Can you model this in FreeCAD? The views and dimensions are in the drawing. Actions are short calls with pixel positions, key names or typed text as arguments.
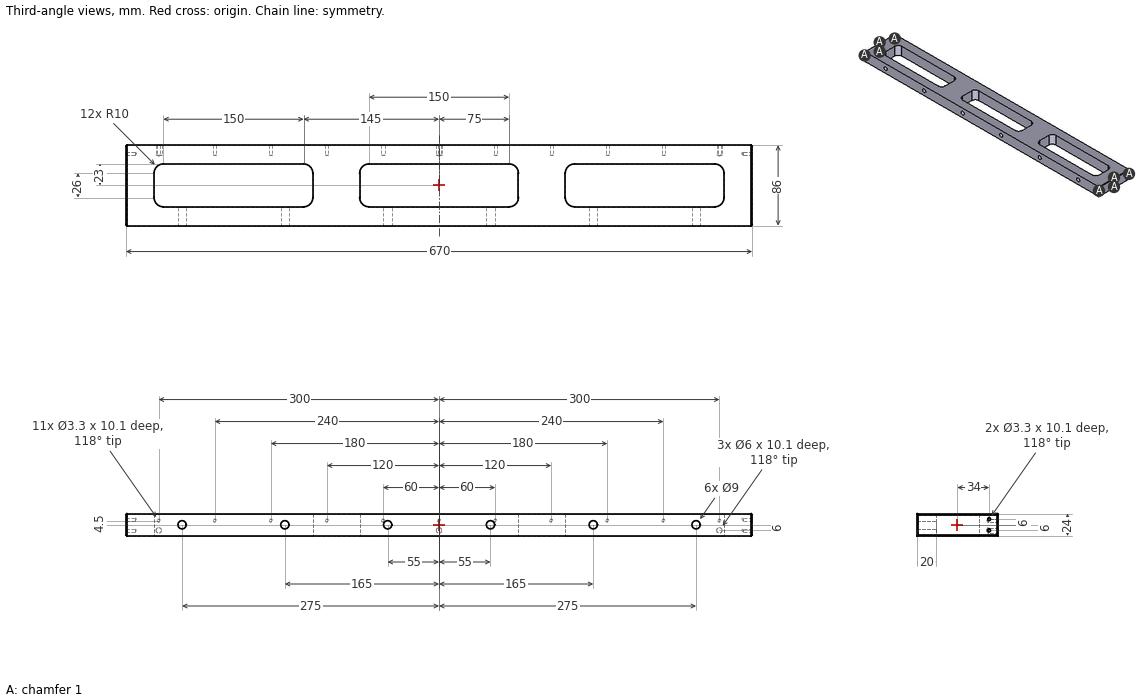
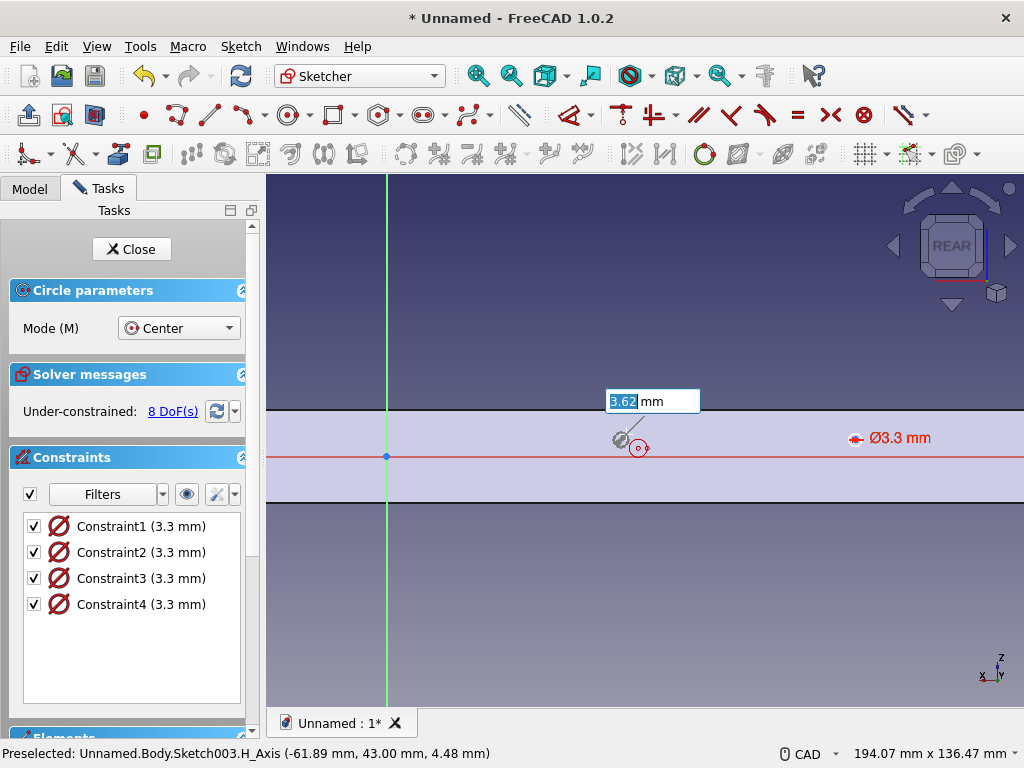
text(3.3)
key(Return)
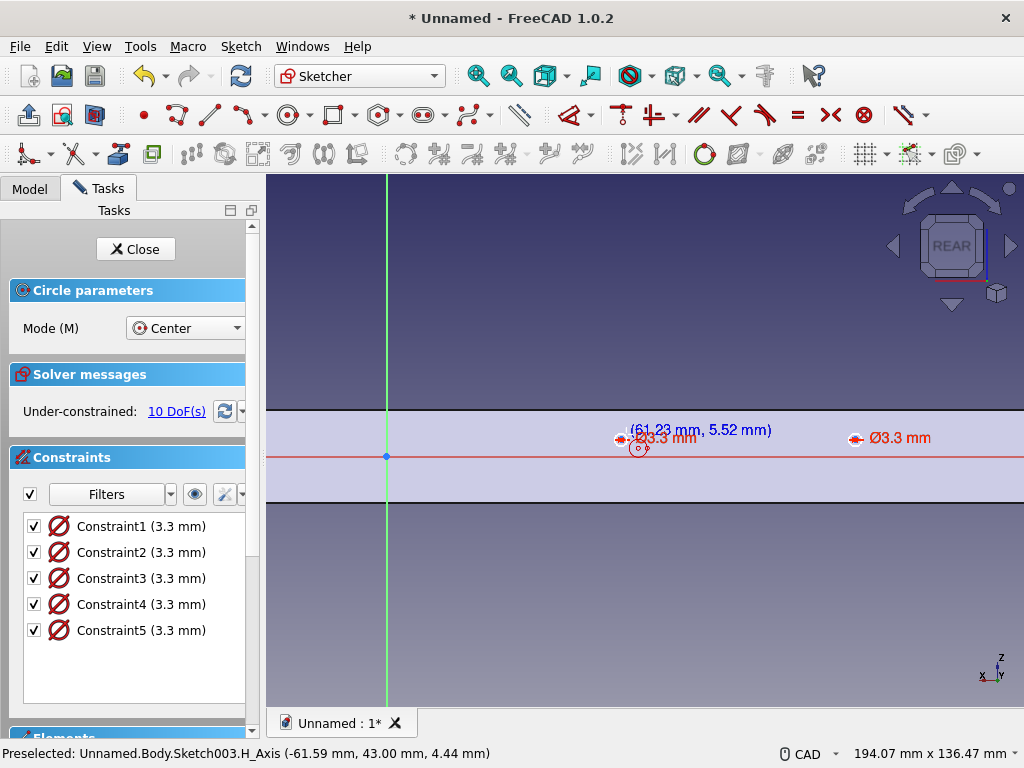
scroll(387, 439, up, 7)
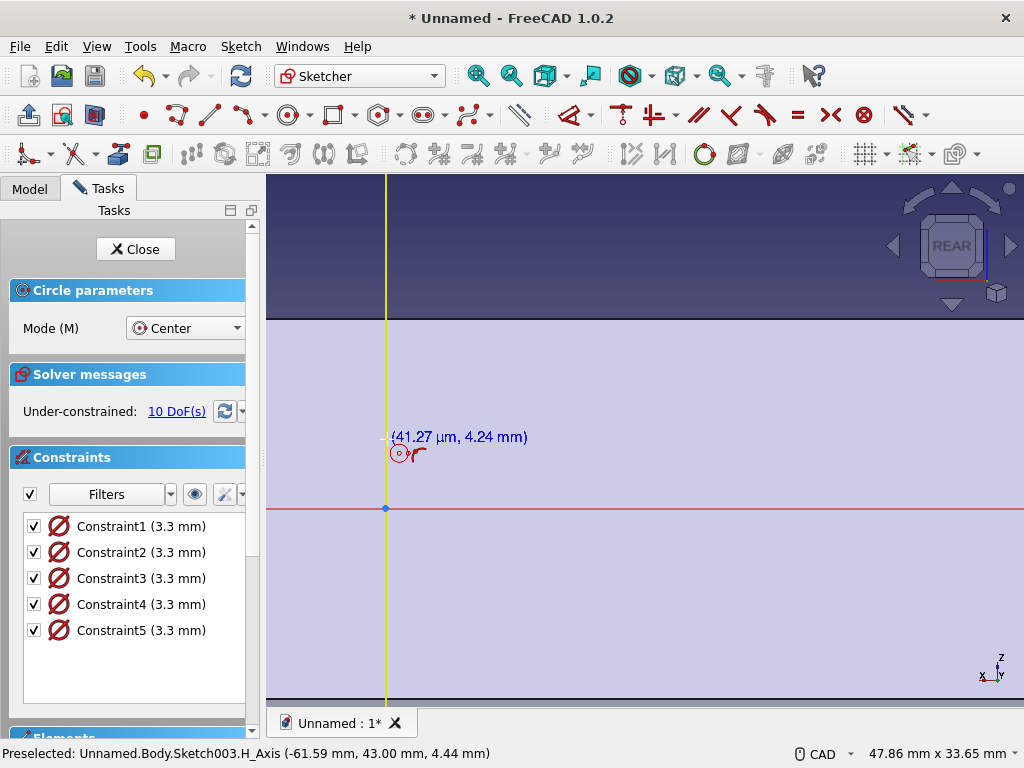
scroll(586, 439, down, 15)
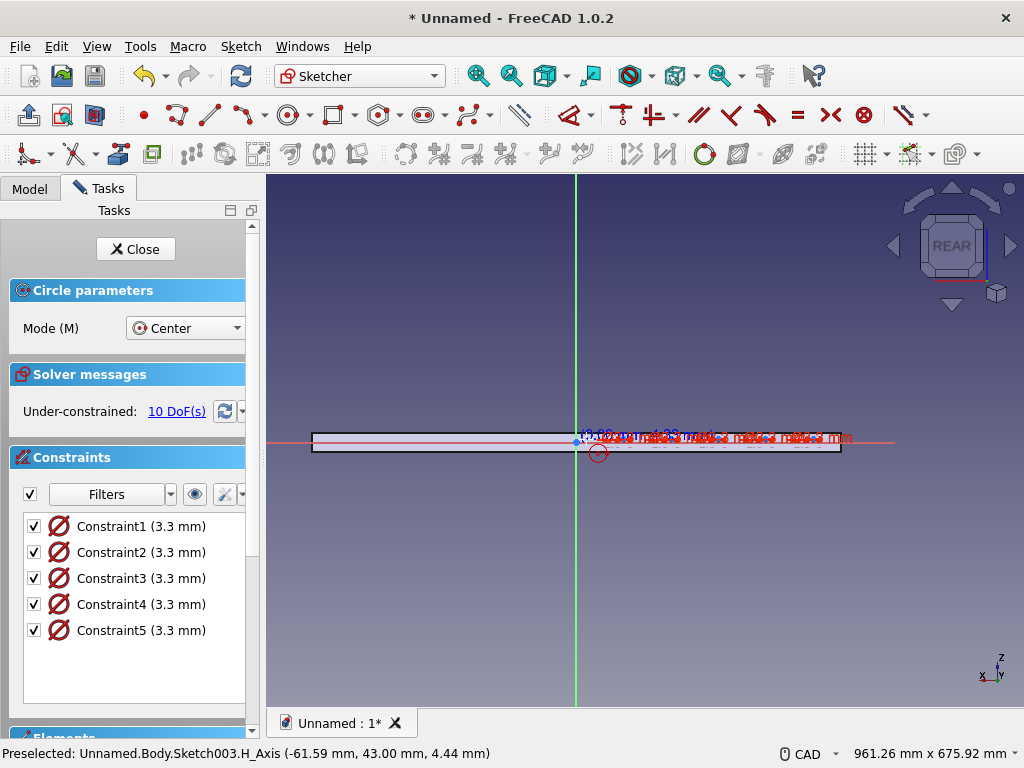
scroll(576, 439, up, 8)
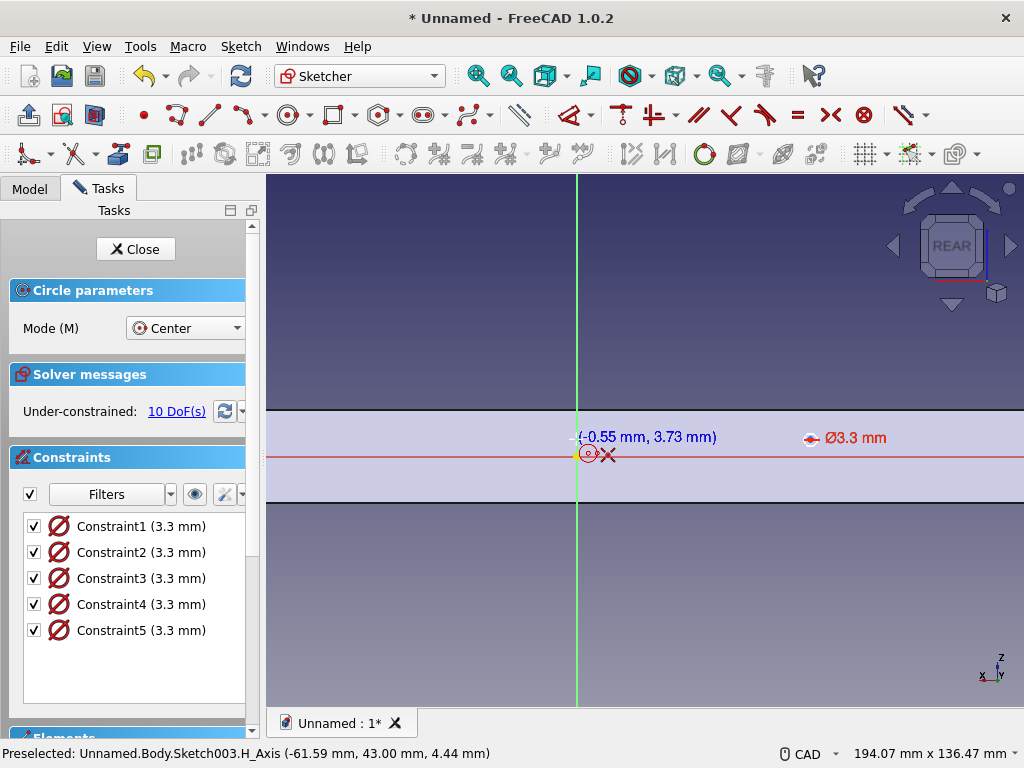
click(577, 439)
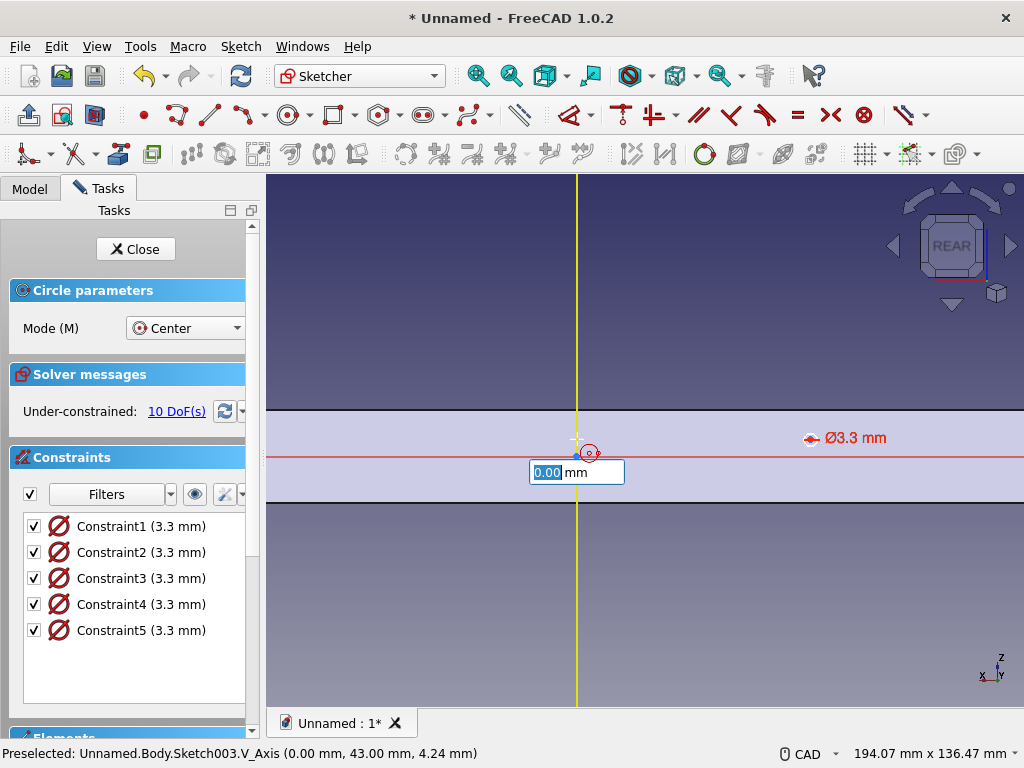
scroll(583, 437, up, 5)
move(581, 436)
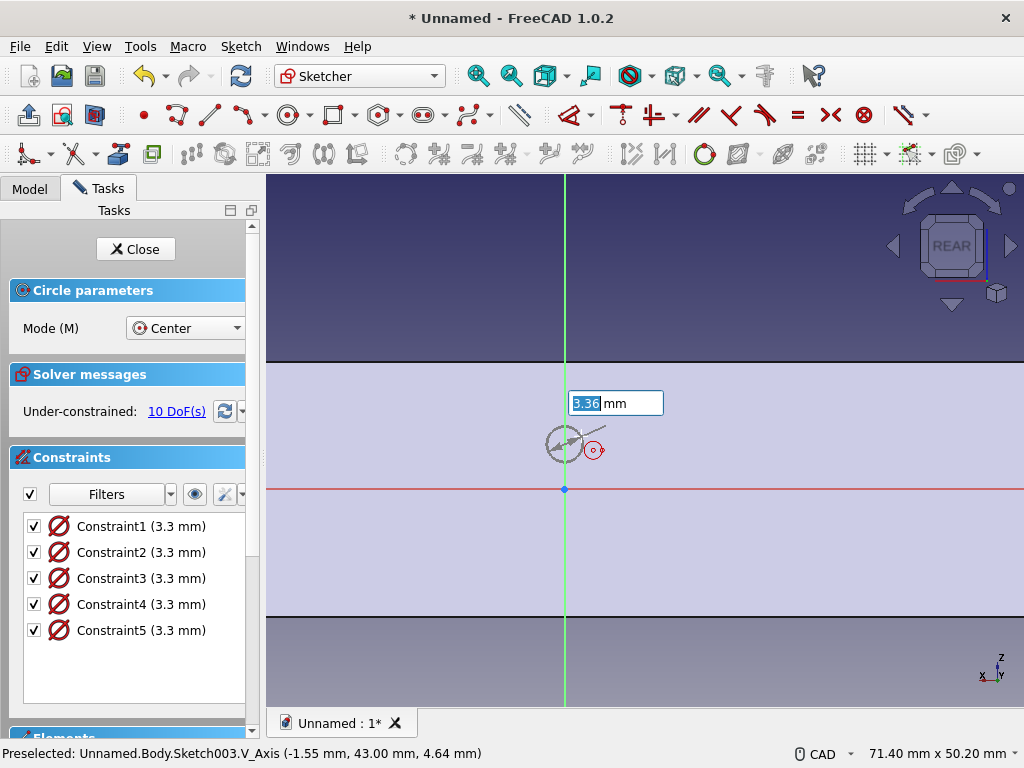
text(3.3)
key(Return)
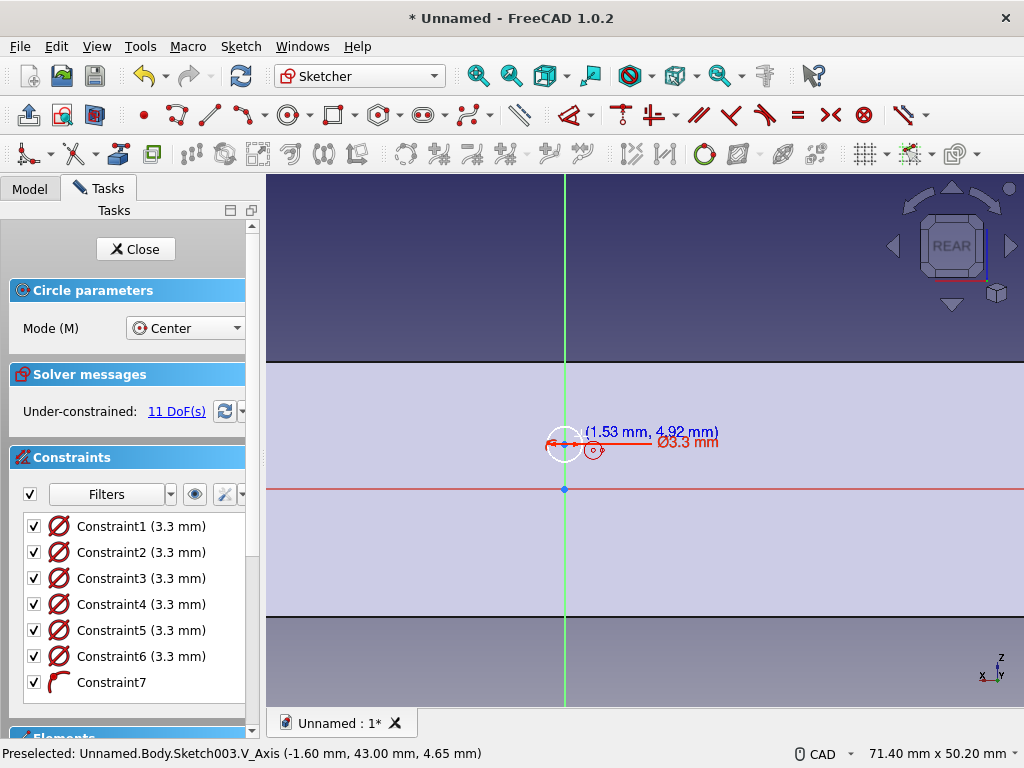
scroll(577, 439, down, 14)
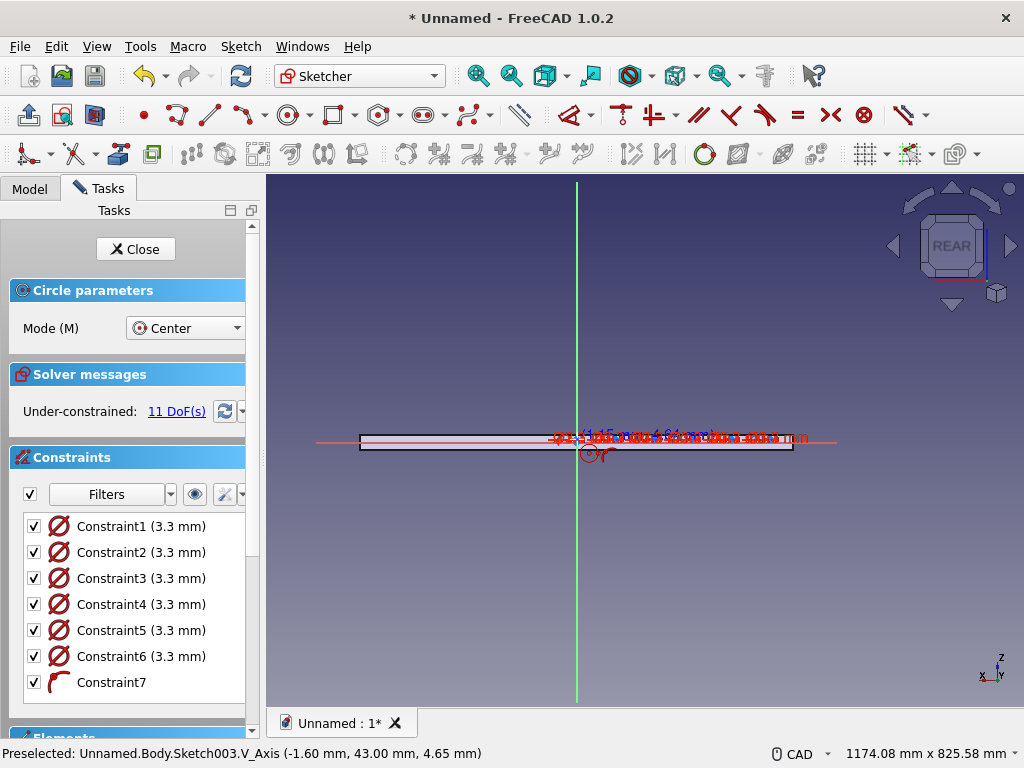
scroll(538, 440, up, 16)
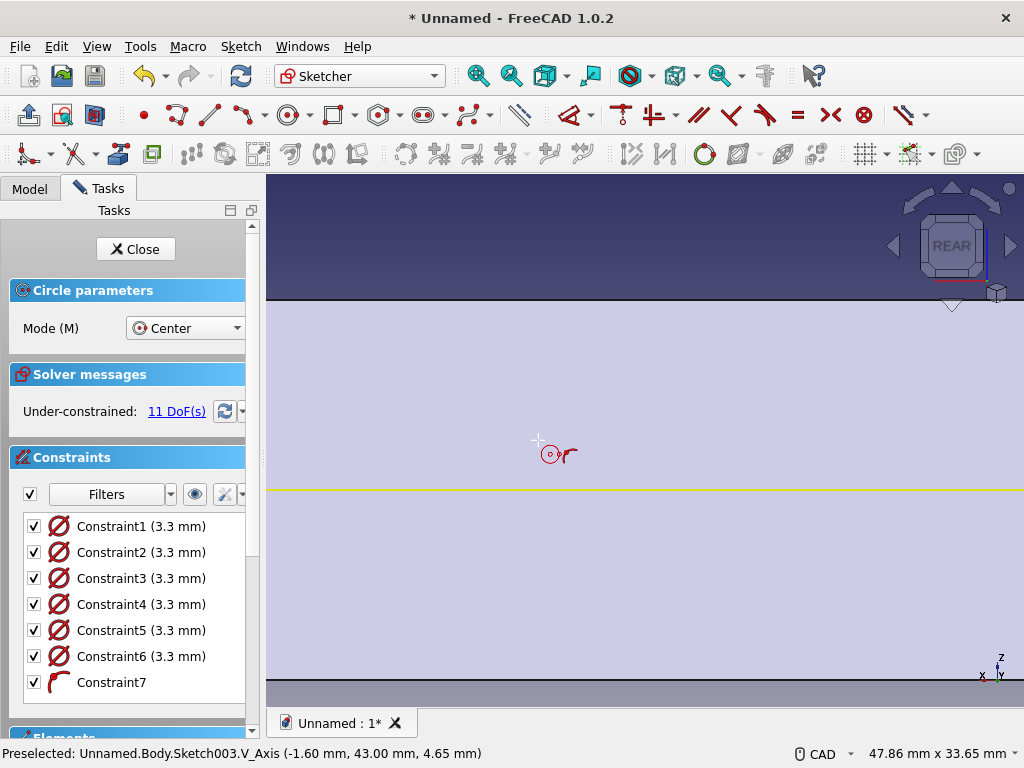
scroll(529, 440, down, 15)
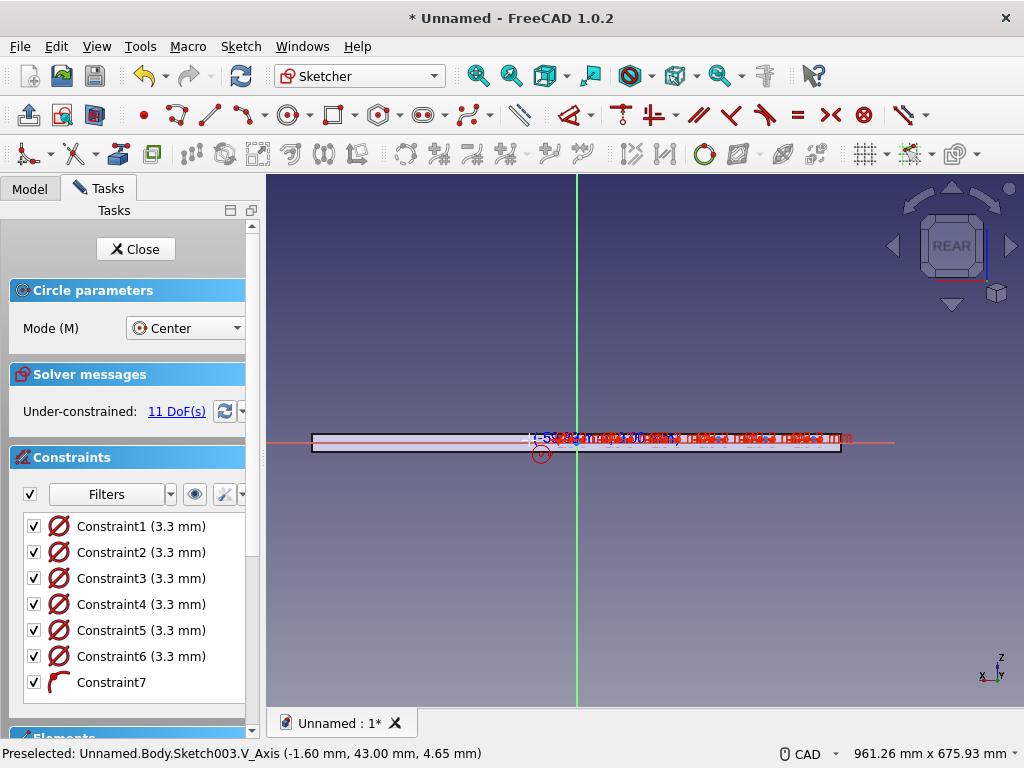
scroll(529, 439, up, 8)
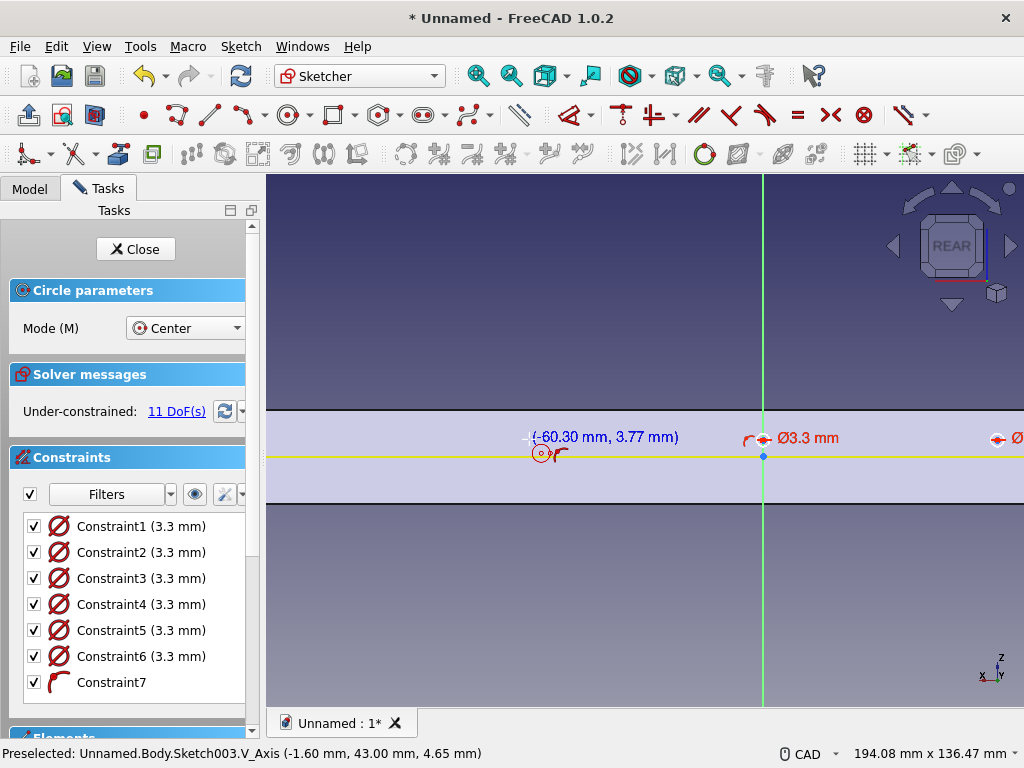
click(529, 439)
move(533, 435)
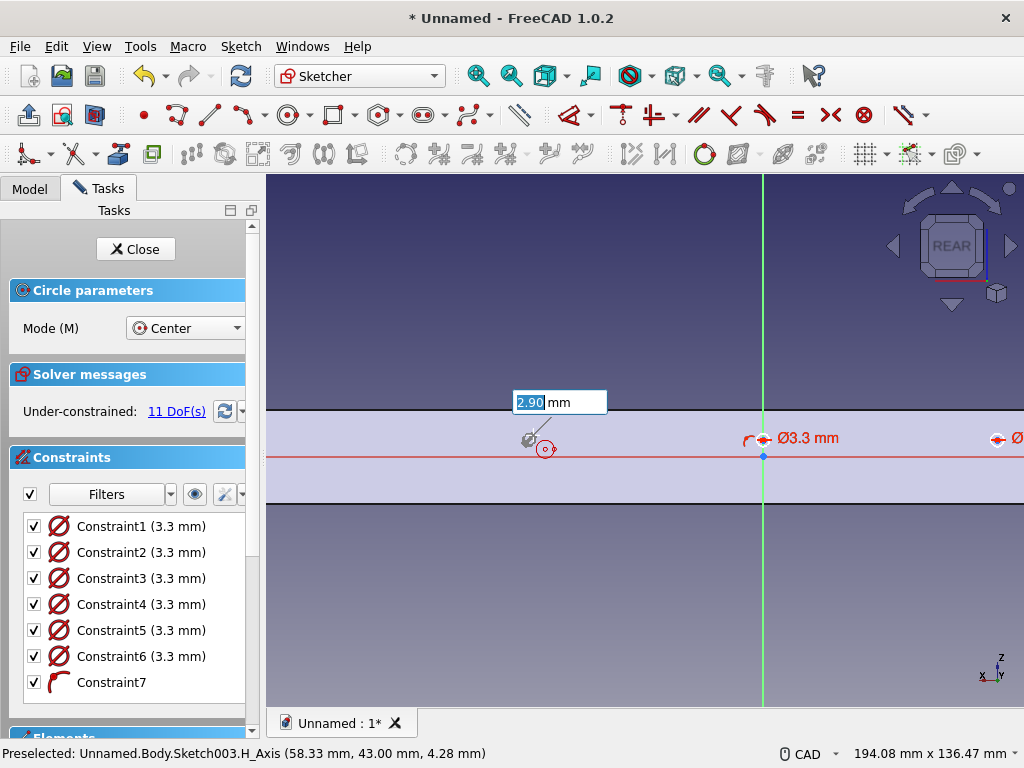
text(3.3)
key(Return)